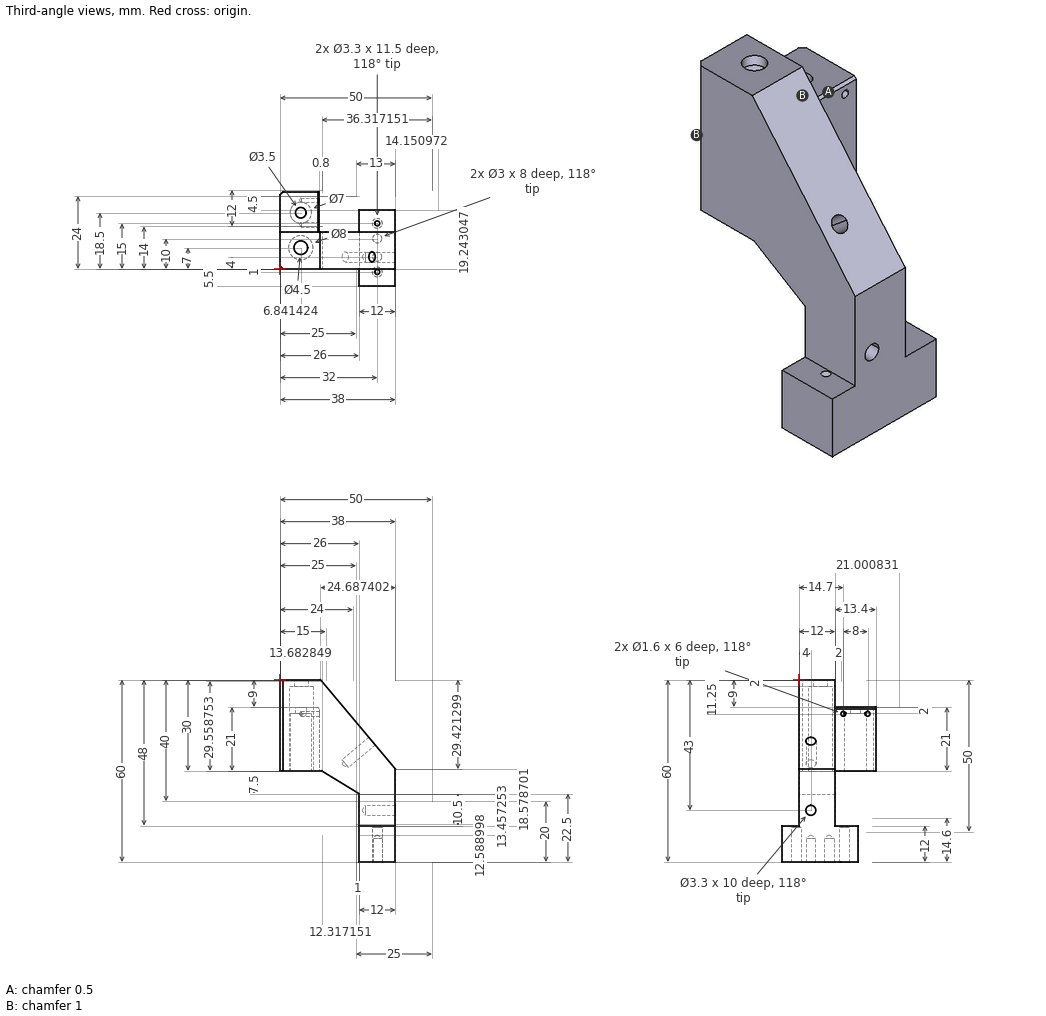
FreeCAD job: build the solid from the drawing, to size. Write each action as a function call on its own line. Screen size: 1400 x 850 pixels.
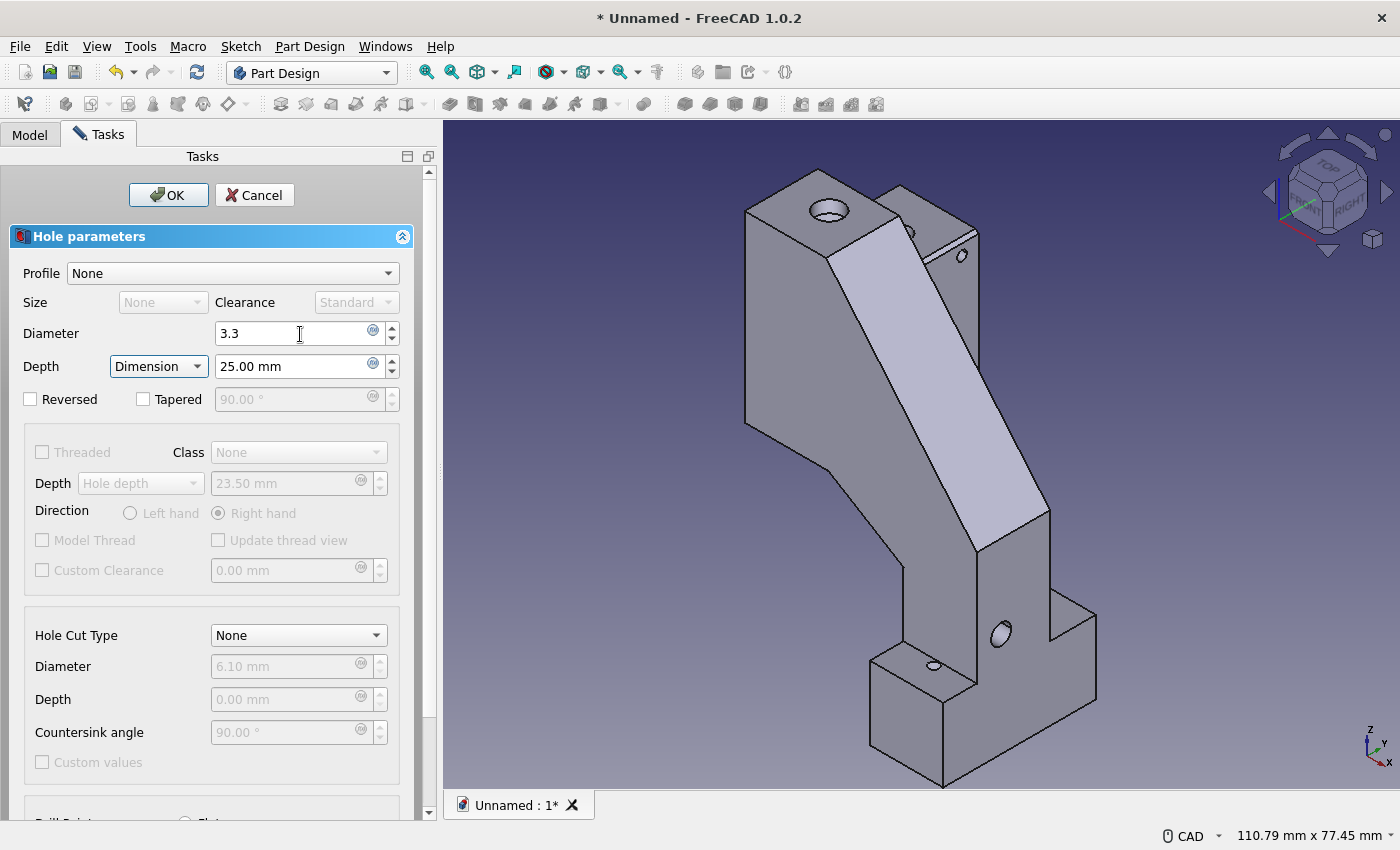
triple_click(300, 366)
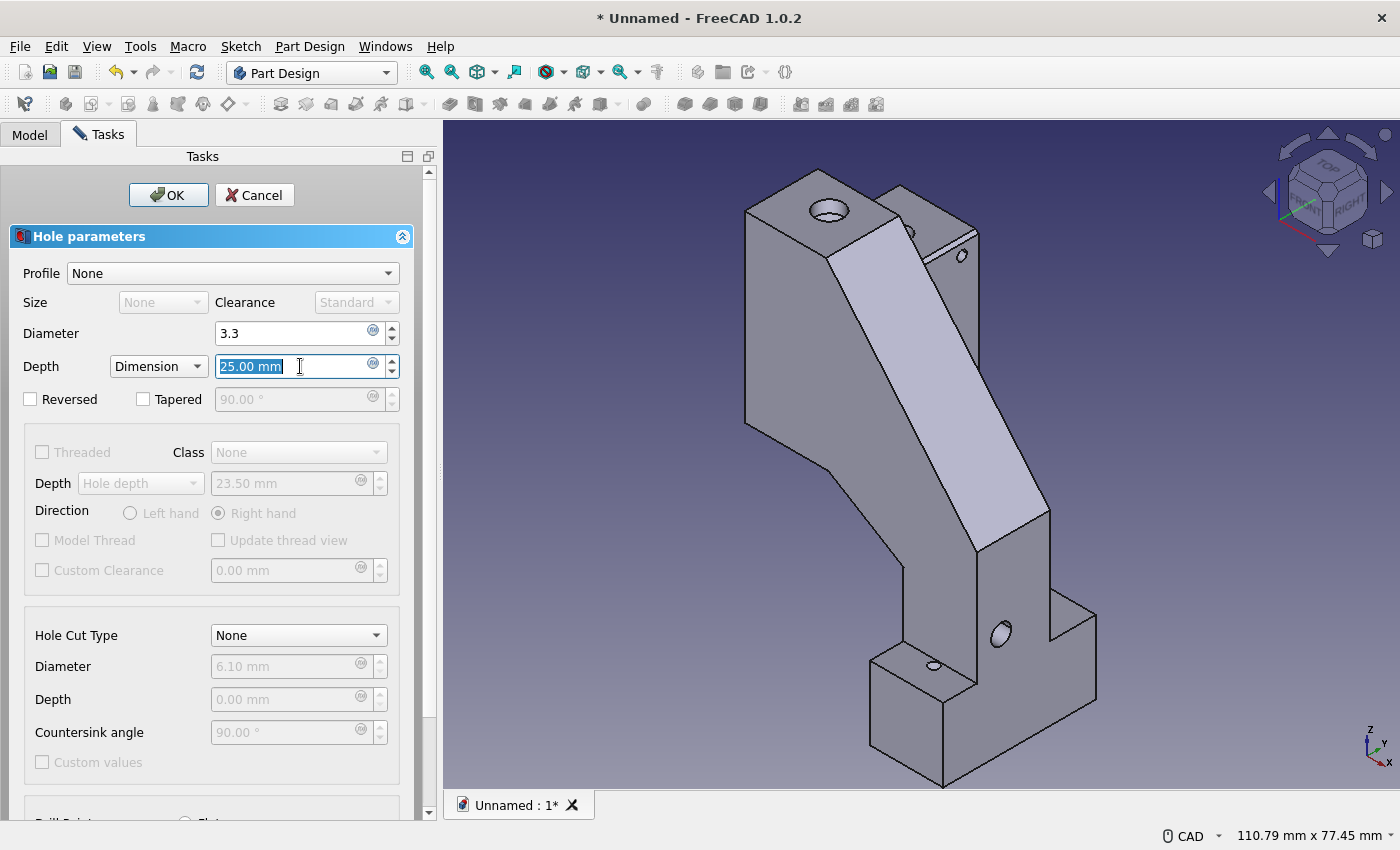
text(10)
key(Tab)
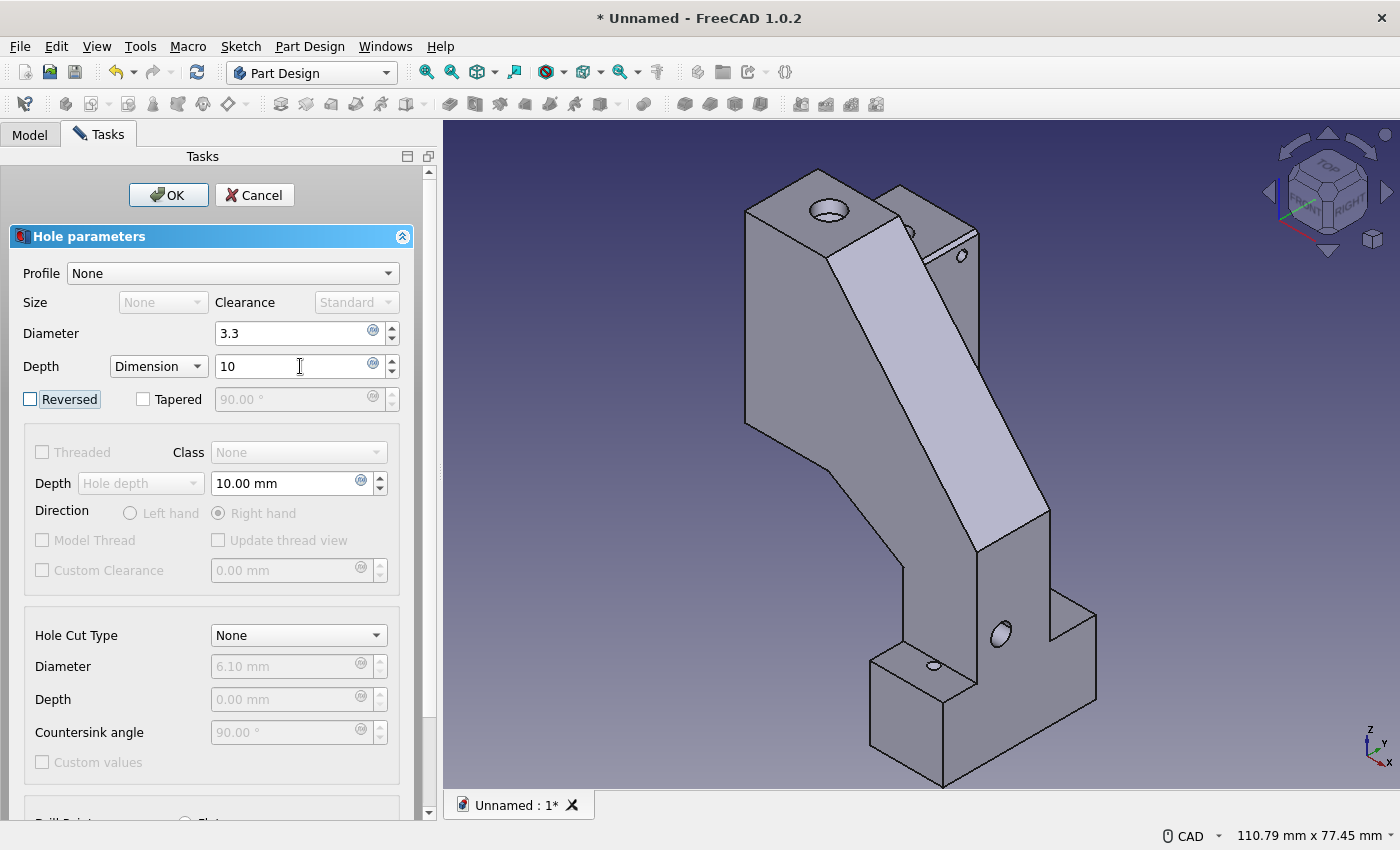
click(169, 195)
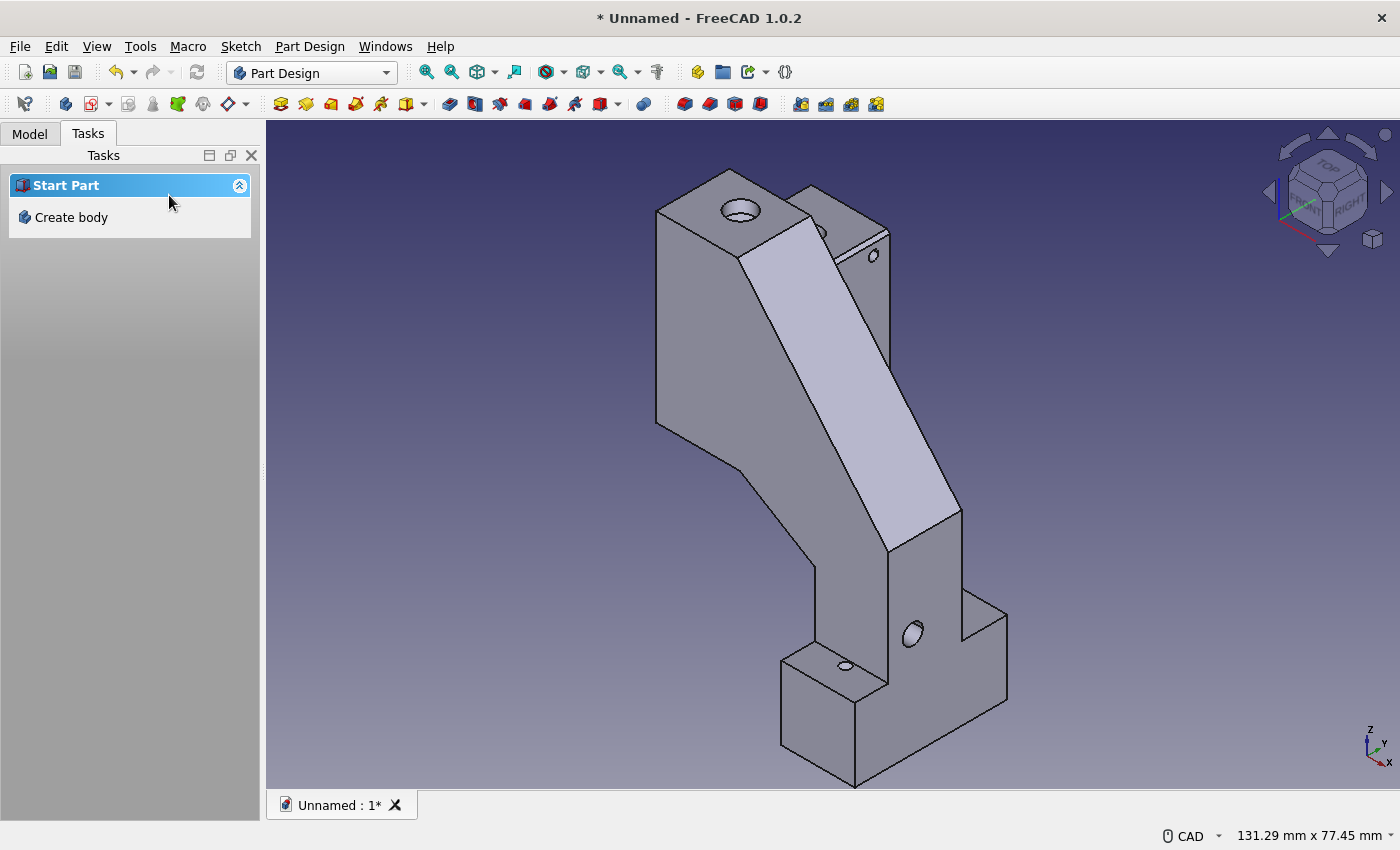
click(893, 467)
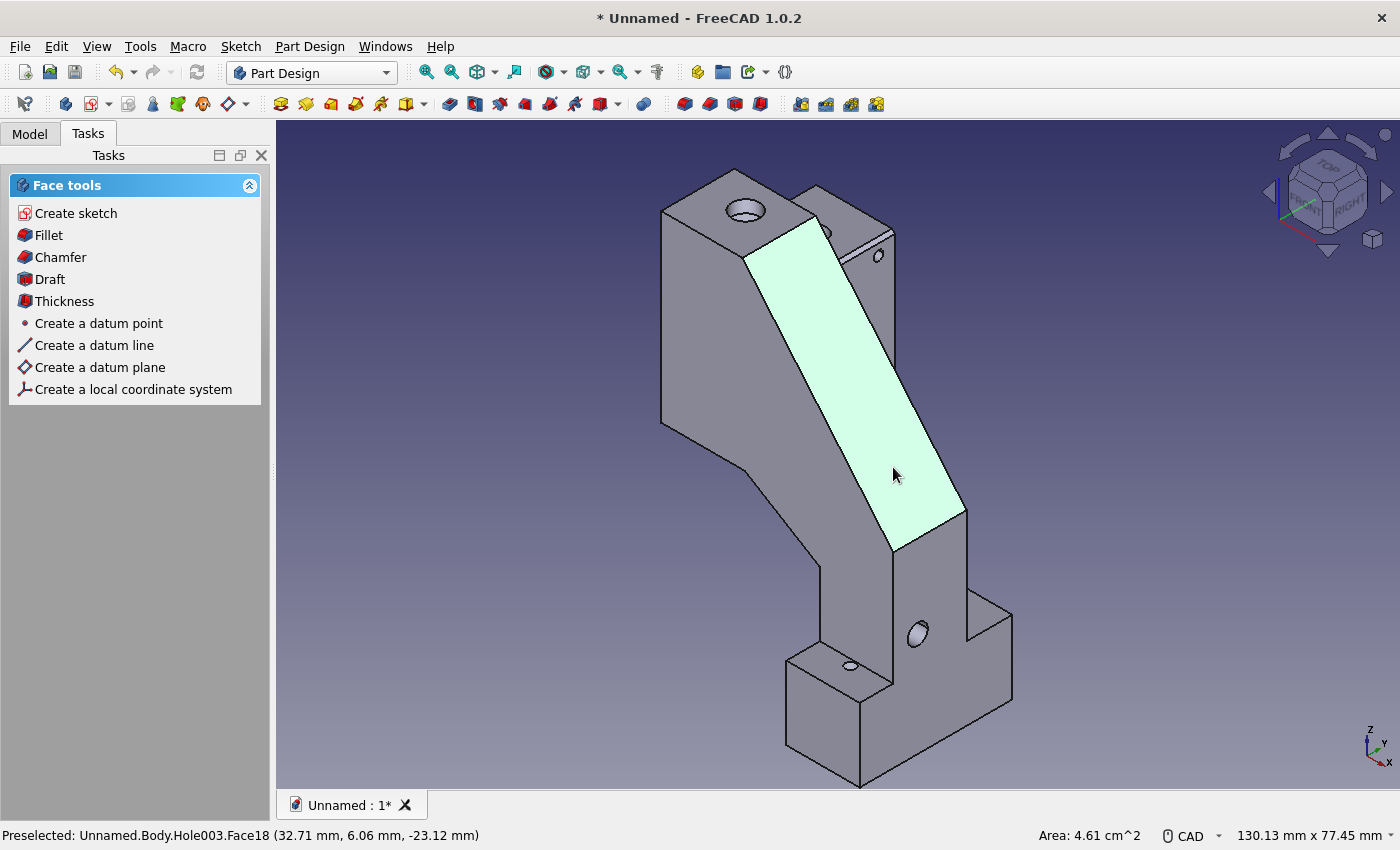
click(90, 104)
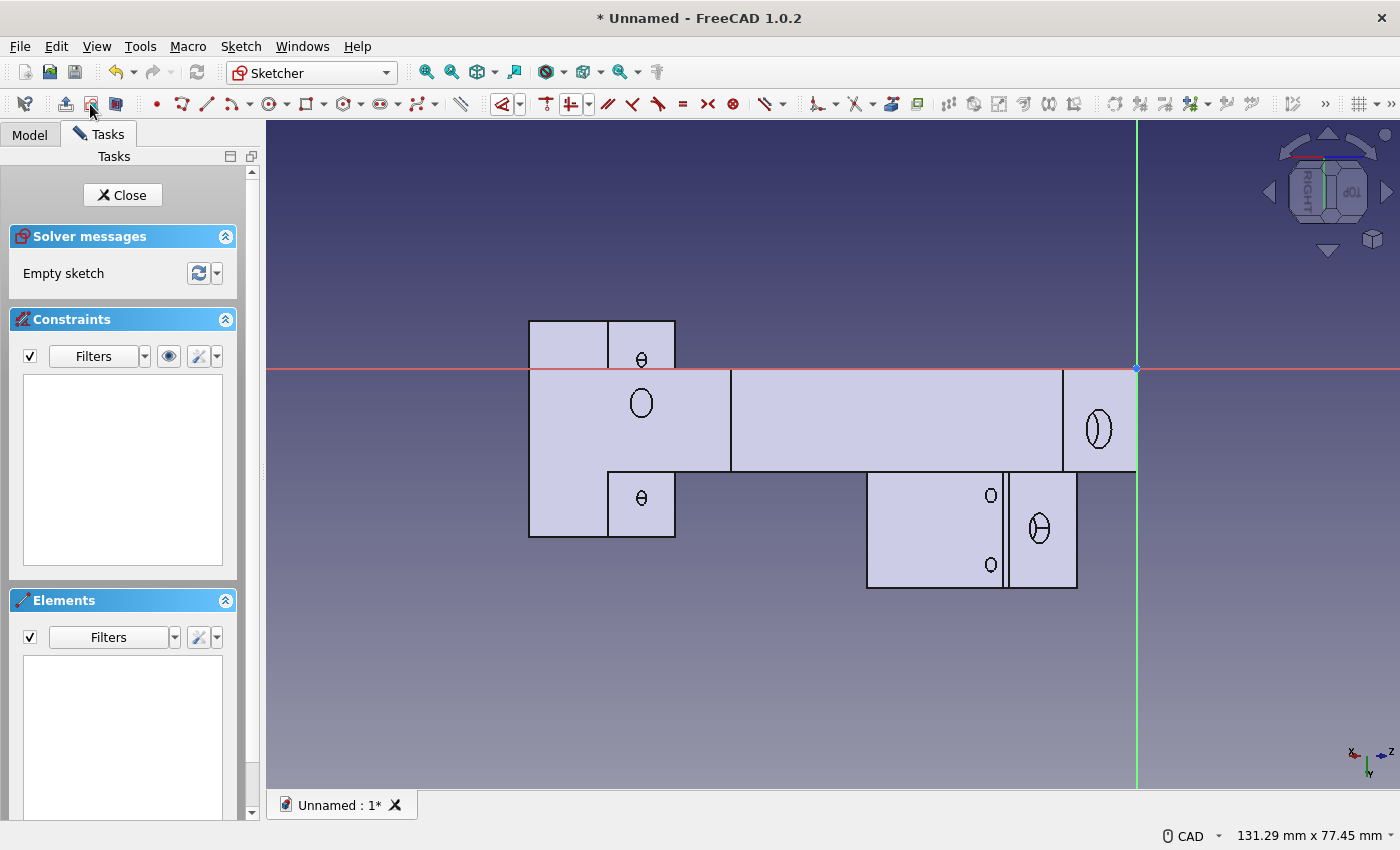
scroll(840, 400, up, 14)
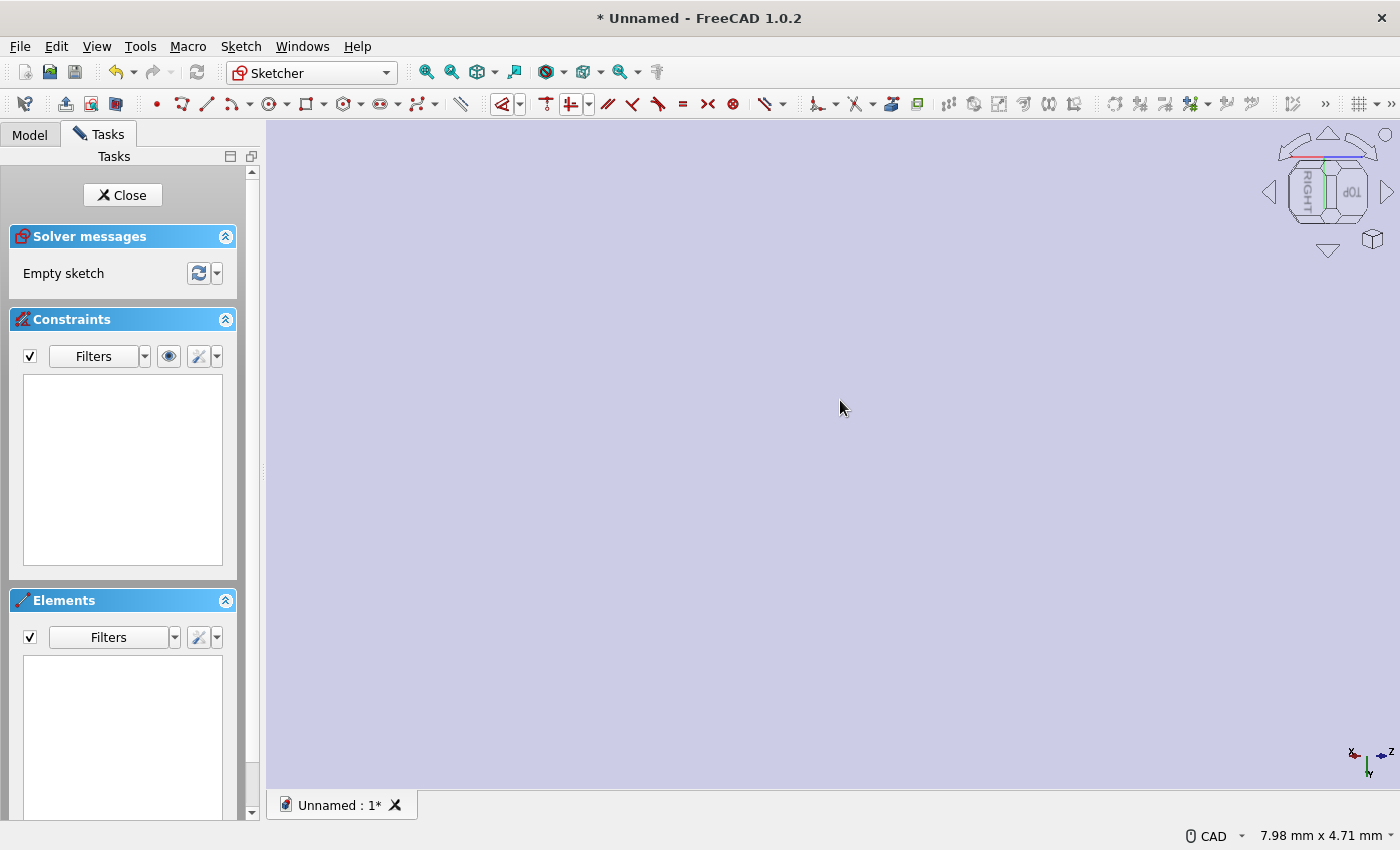
click(268, 104)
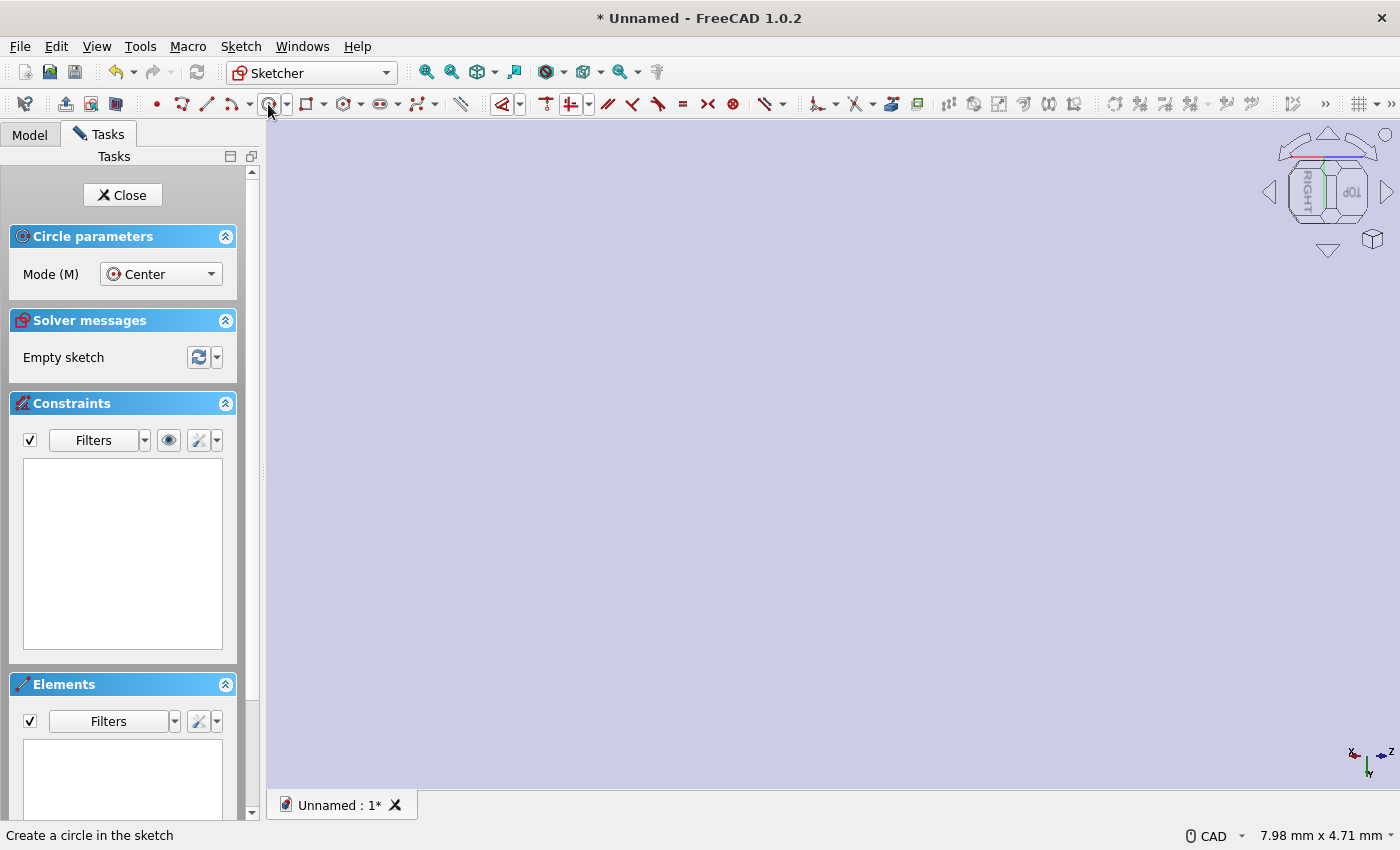
click(750, 445)
click(916, 279)
key(Escape)